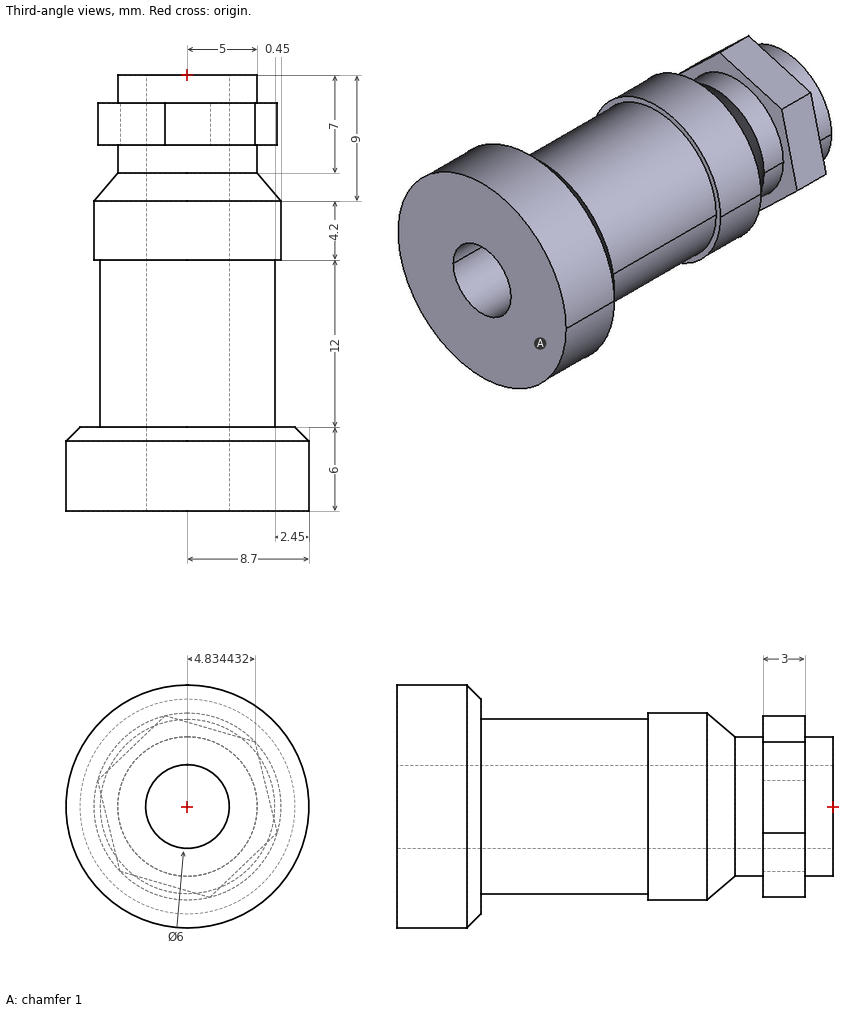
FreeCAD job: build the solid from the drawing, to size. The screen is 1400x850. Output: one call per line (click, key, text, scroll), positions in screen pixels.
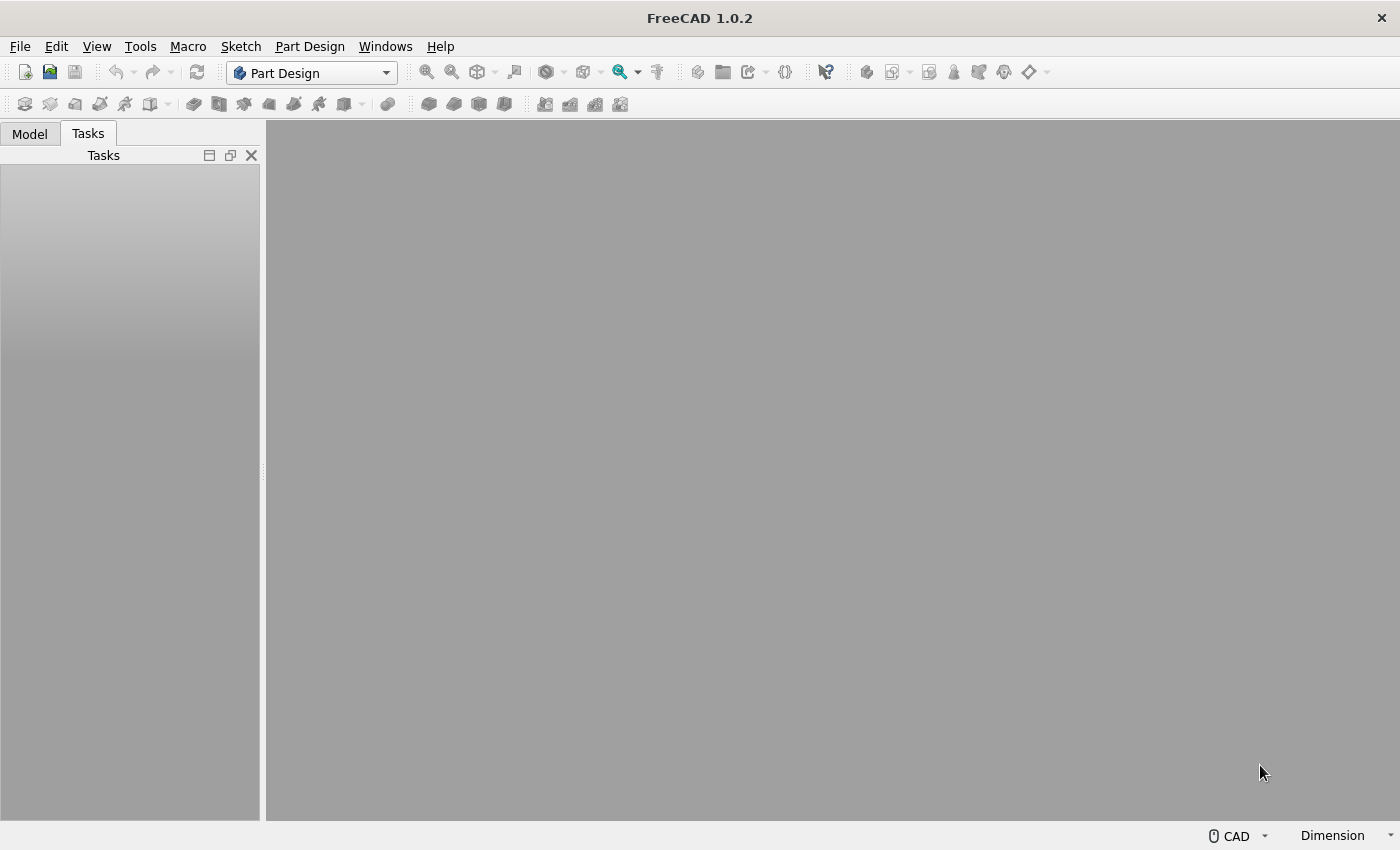
click(25, 72)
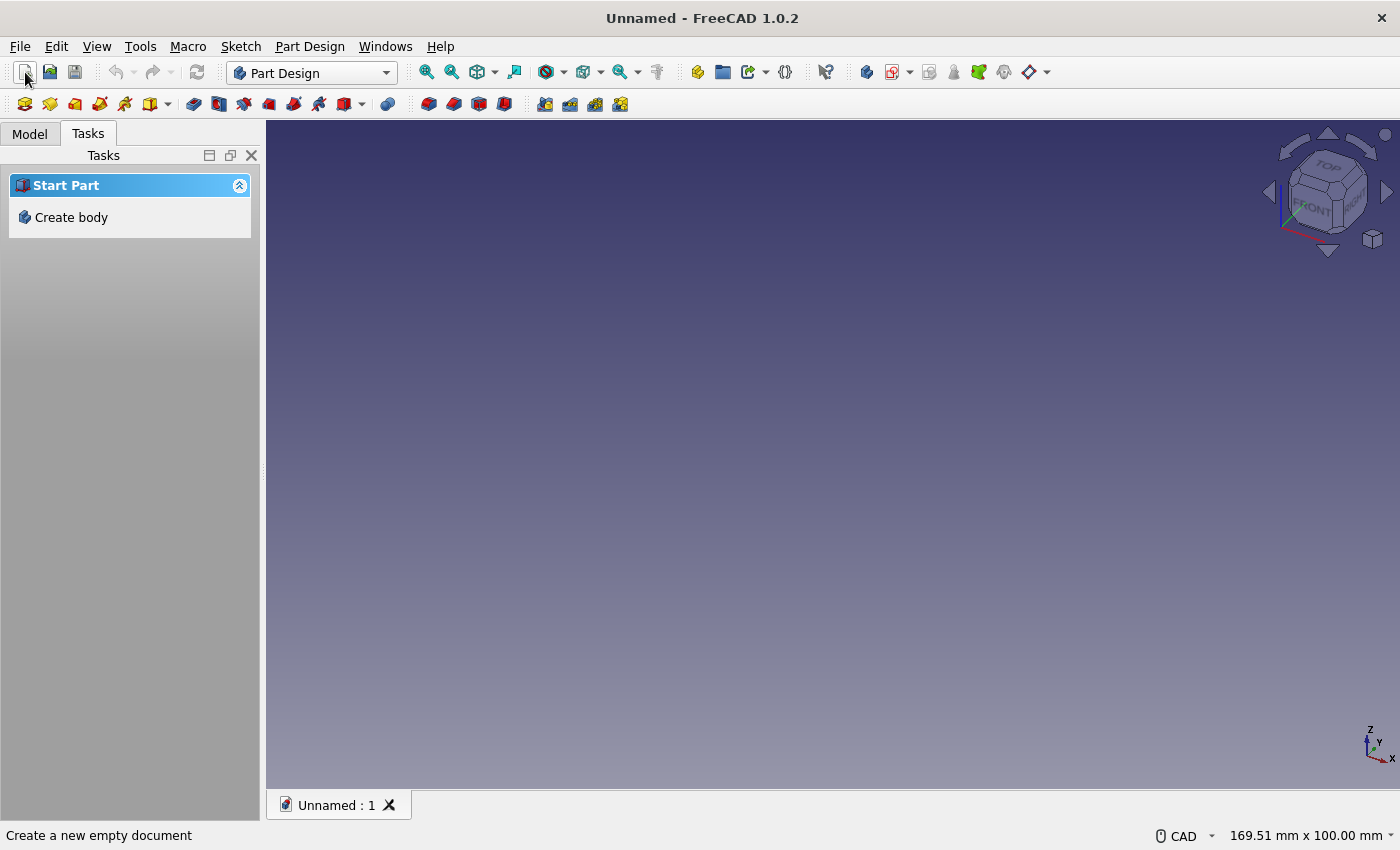
click(892, 72)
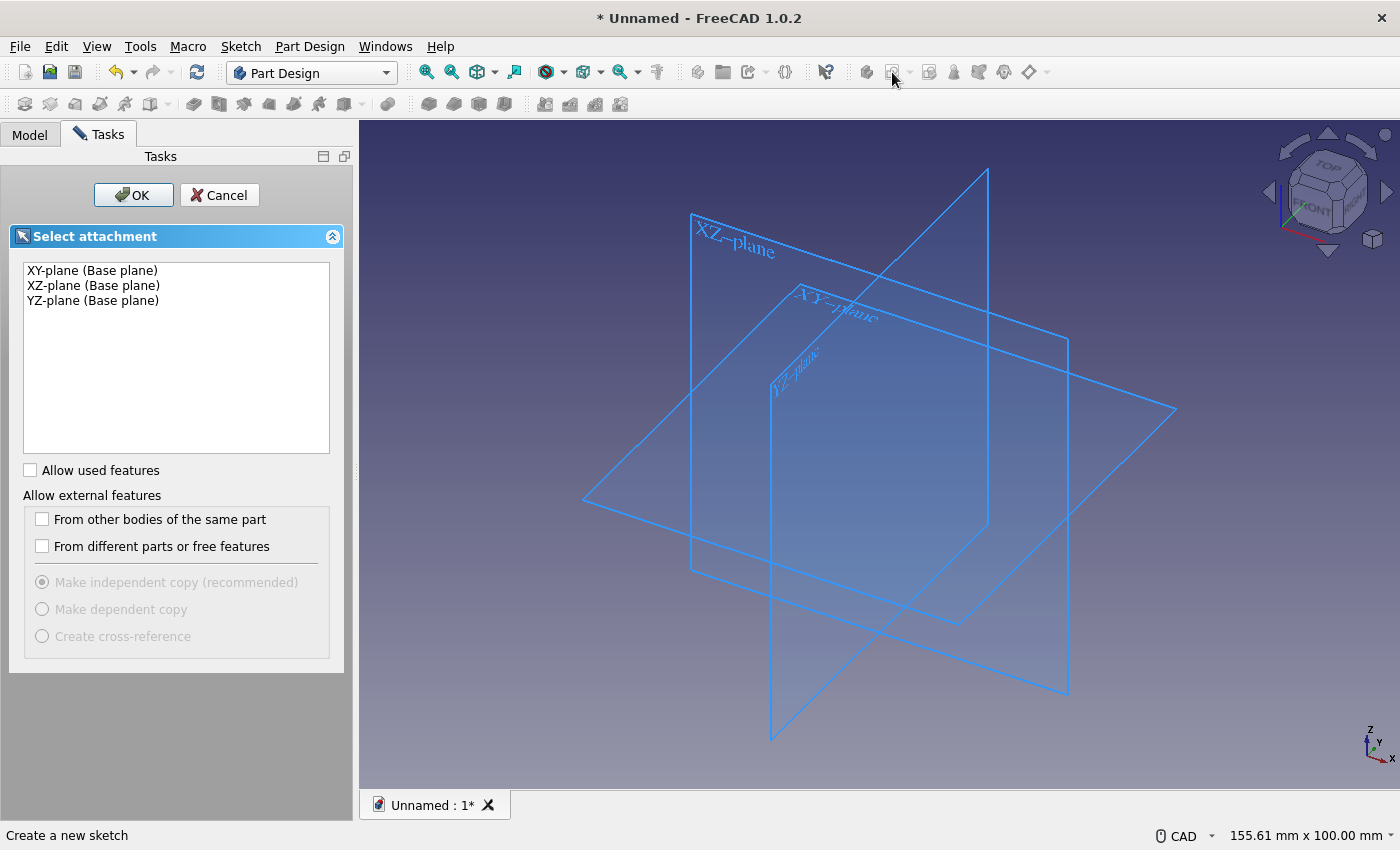
click(84, 270)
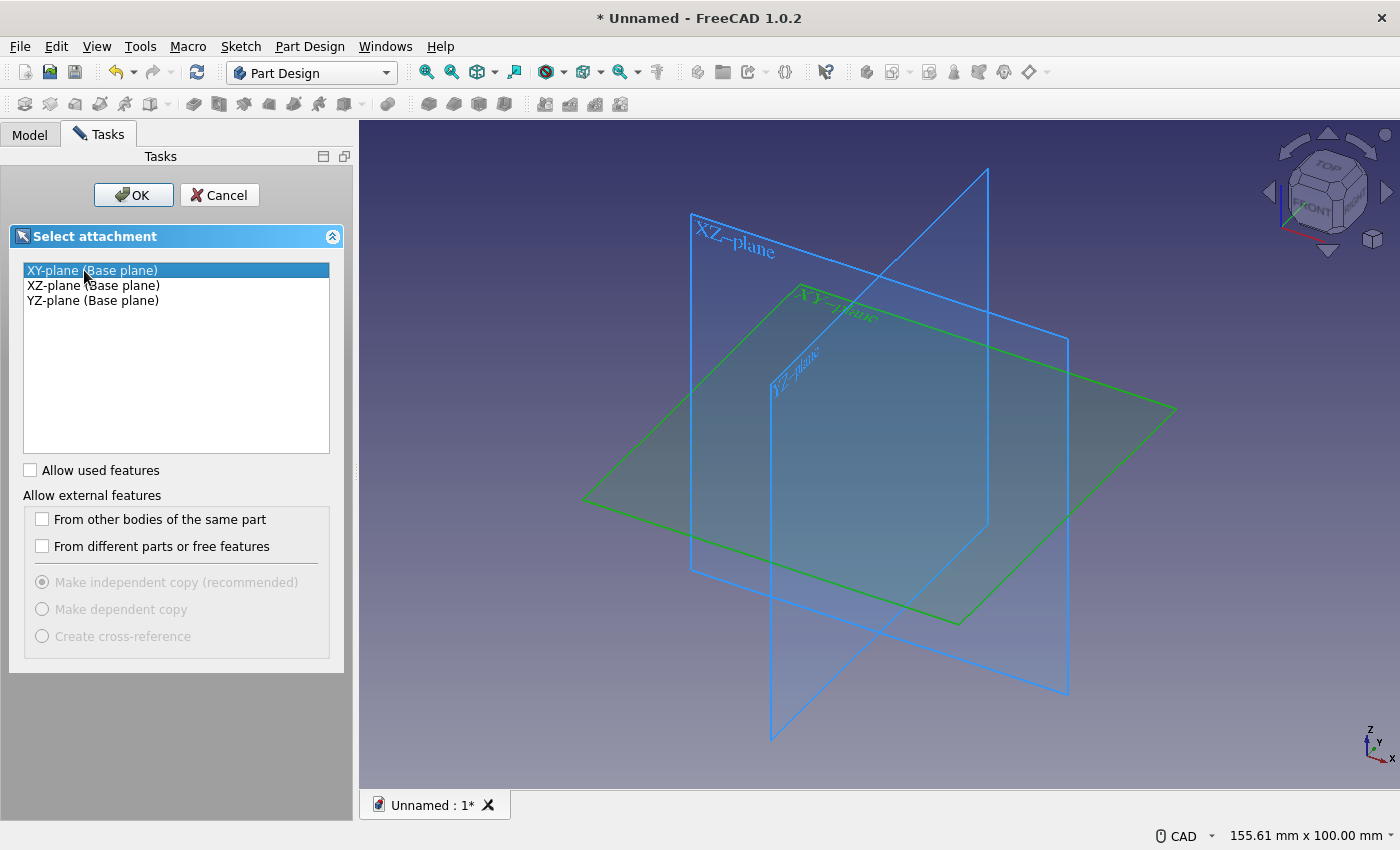
click(134, 195)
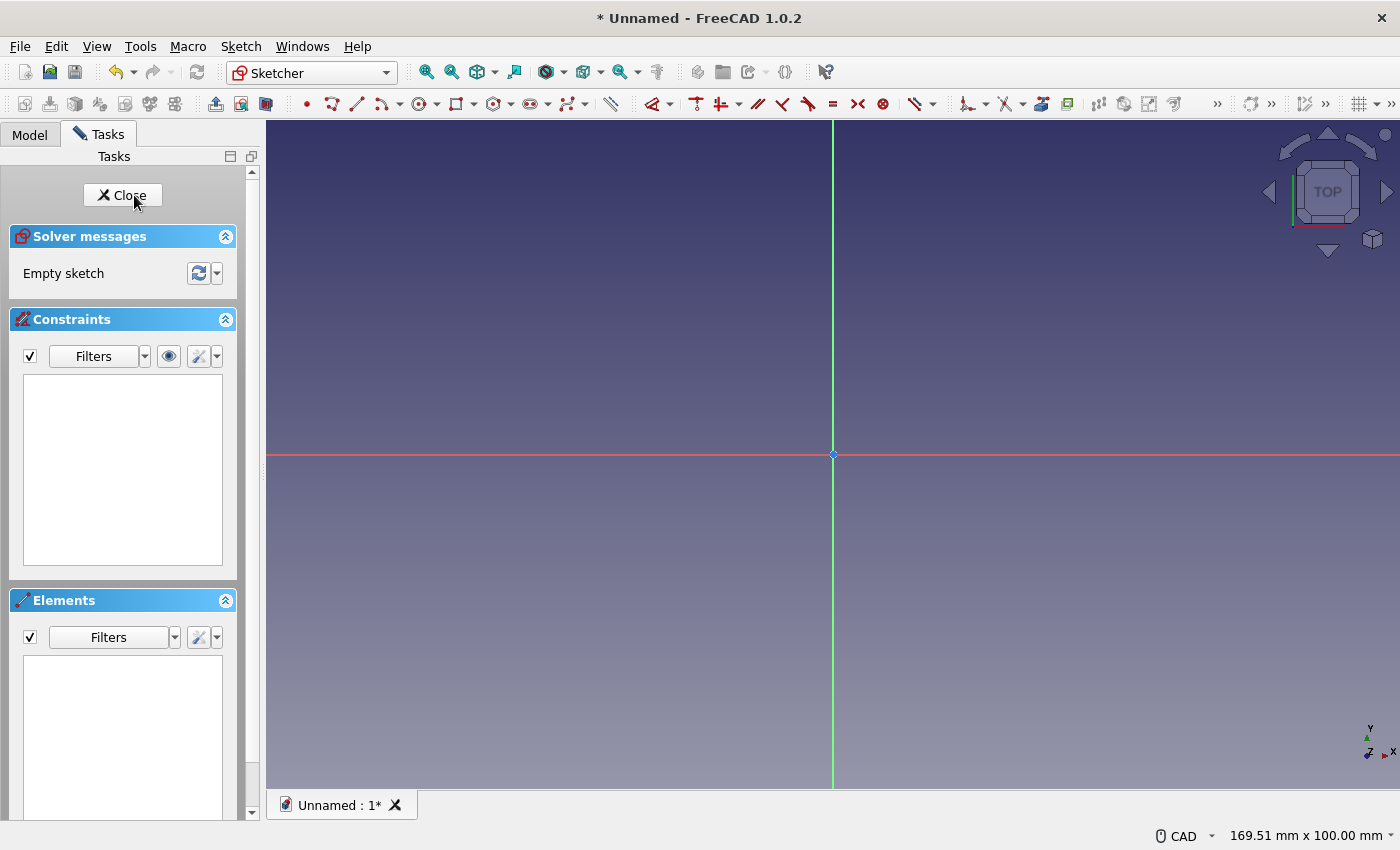
scroll(942, 644, up, 4)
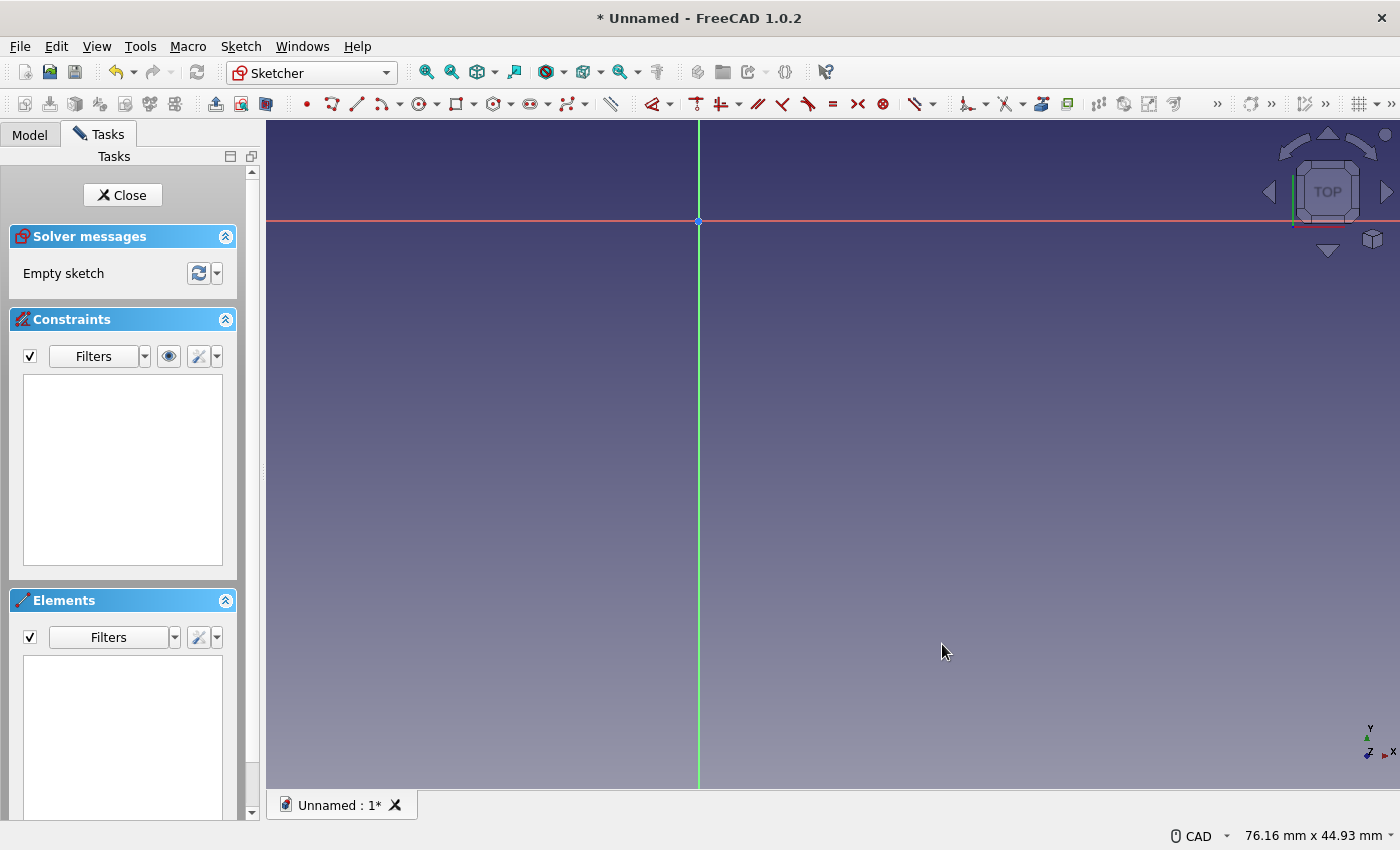
click(332, 104)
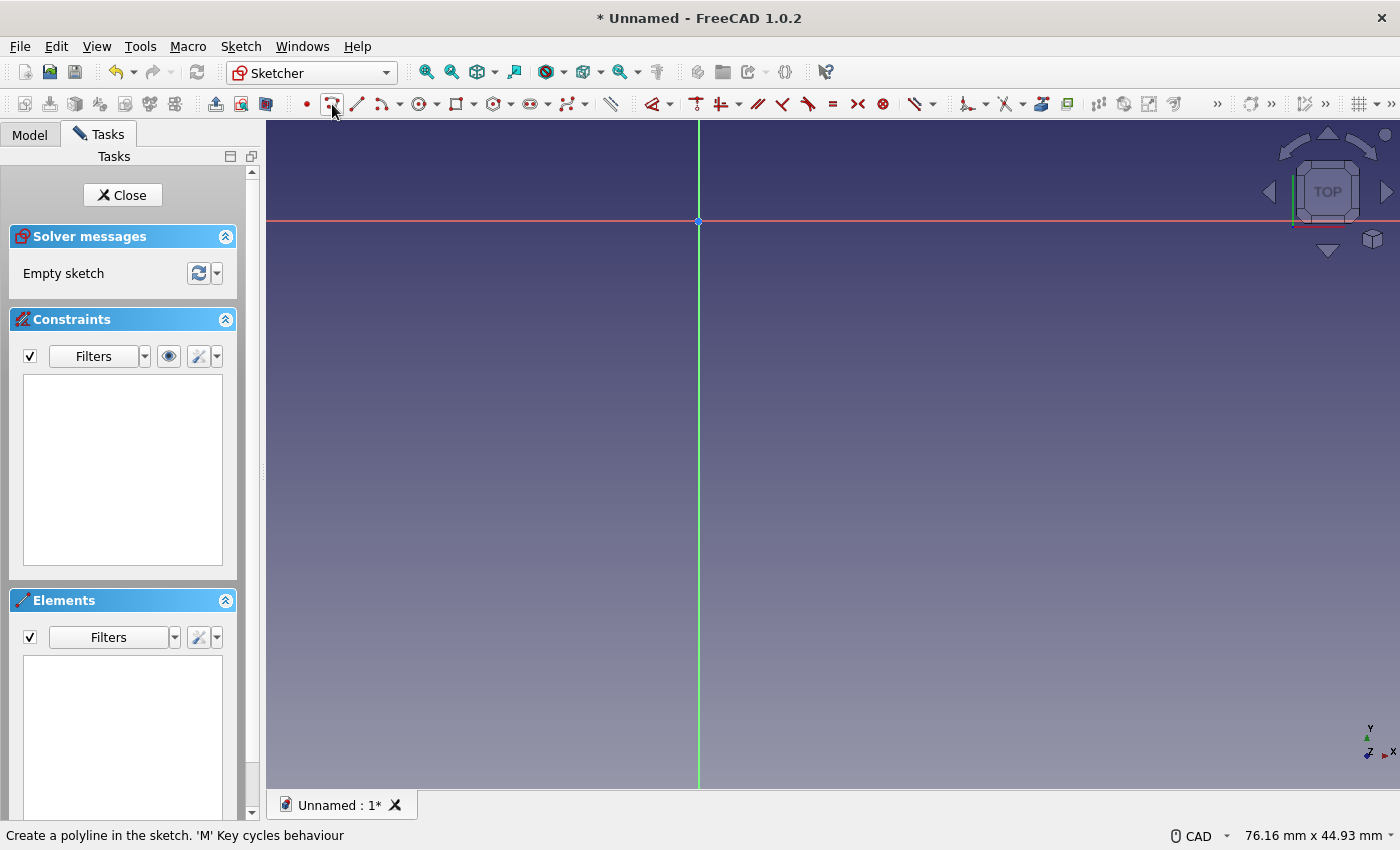
click(699, 221)
click(708, 686)
click(828, 686)
click(828, 596)
click(792, 596)
click(792, 418)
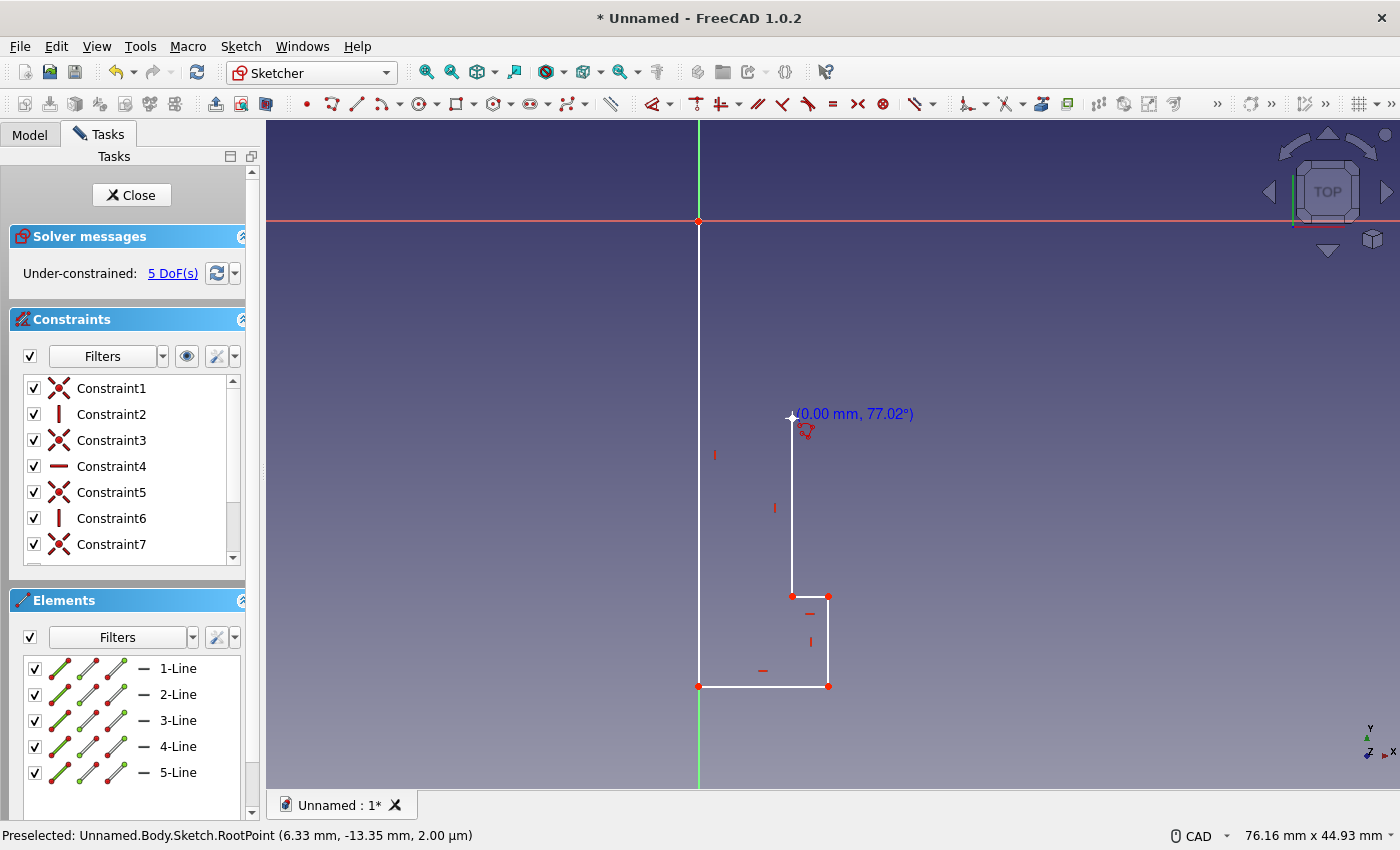
scroll(798, 418, up, 5)